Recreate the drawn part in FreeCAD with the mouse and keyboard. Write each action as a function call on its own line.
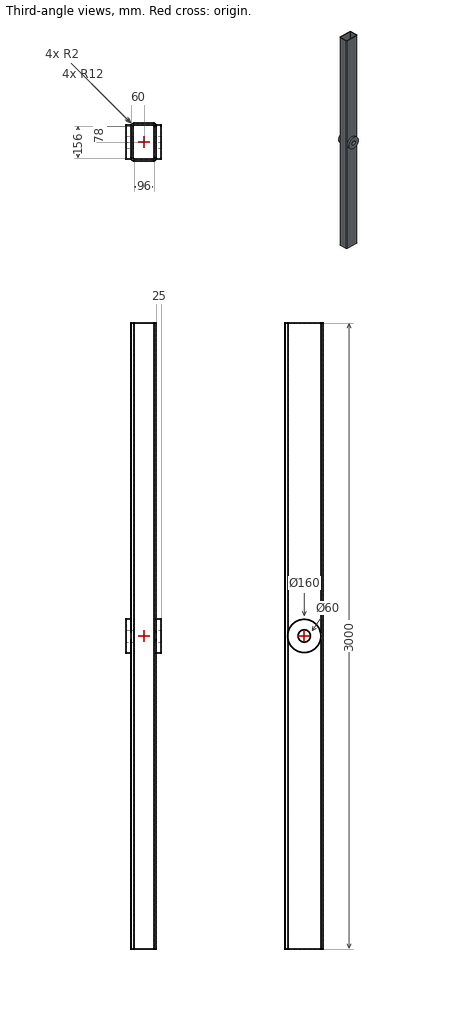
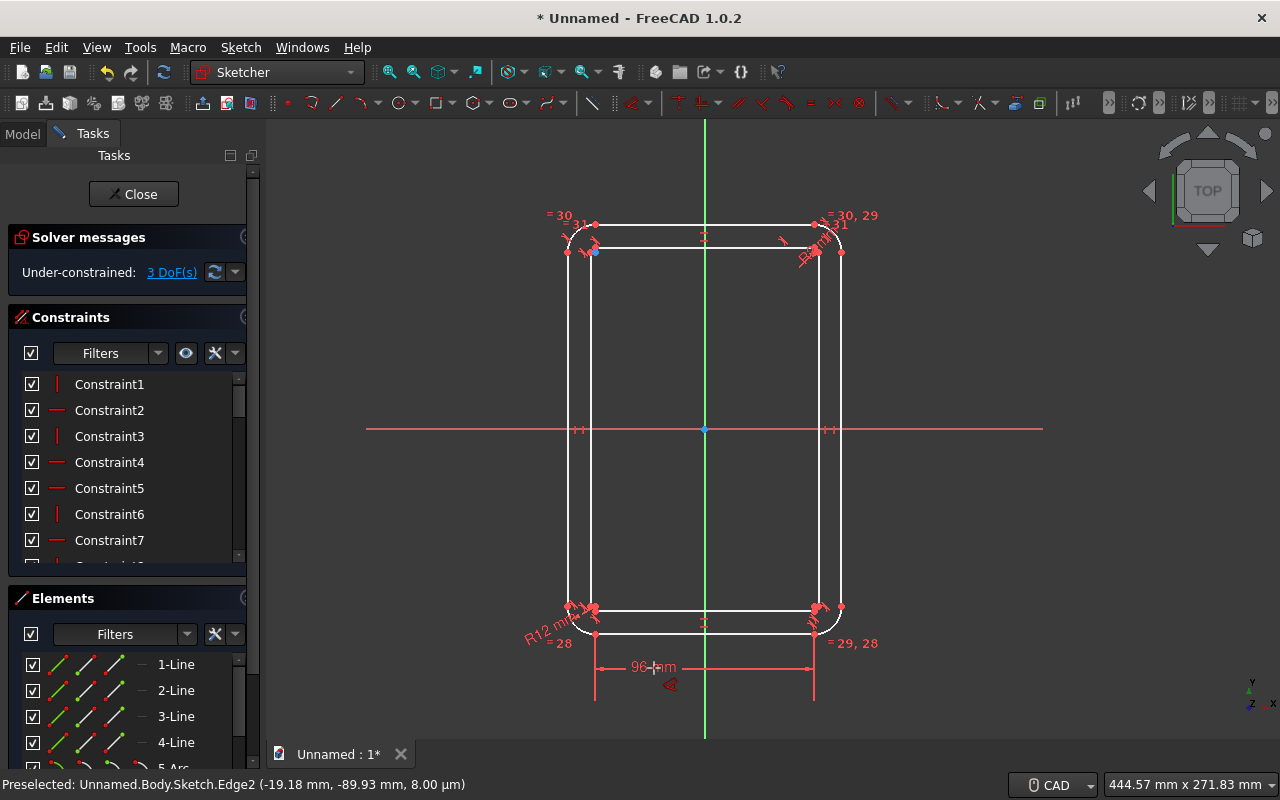
click(568, 359)
click(534, 348)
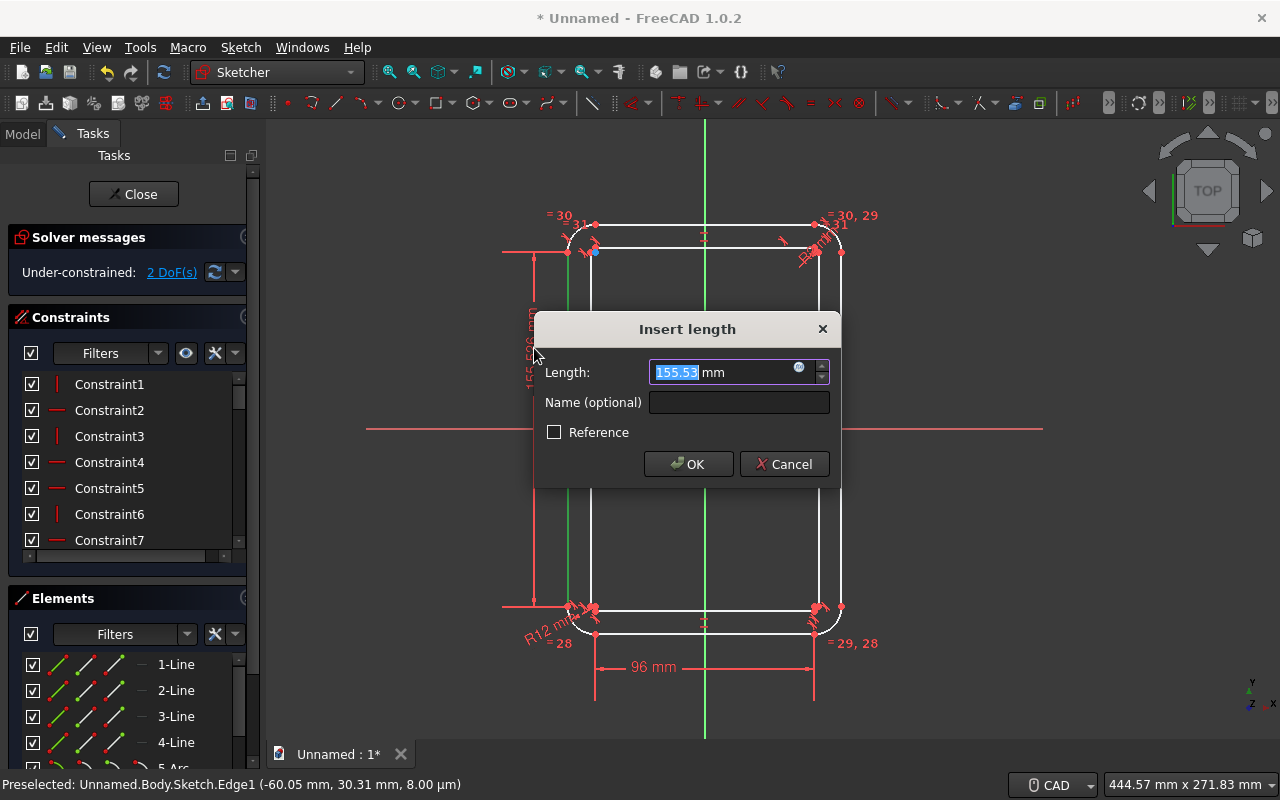
text(156)
key(Return)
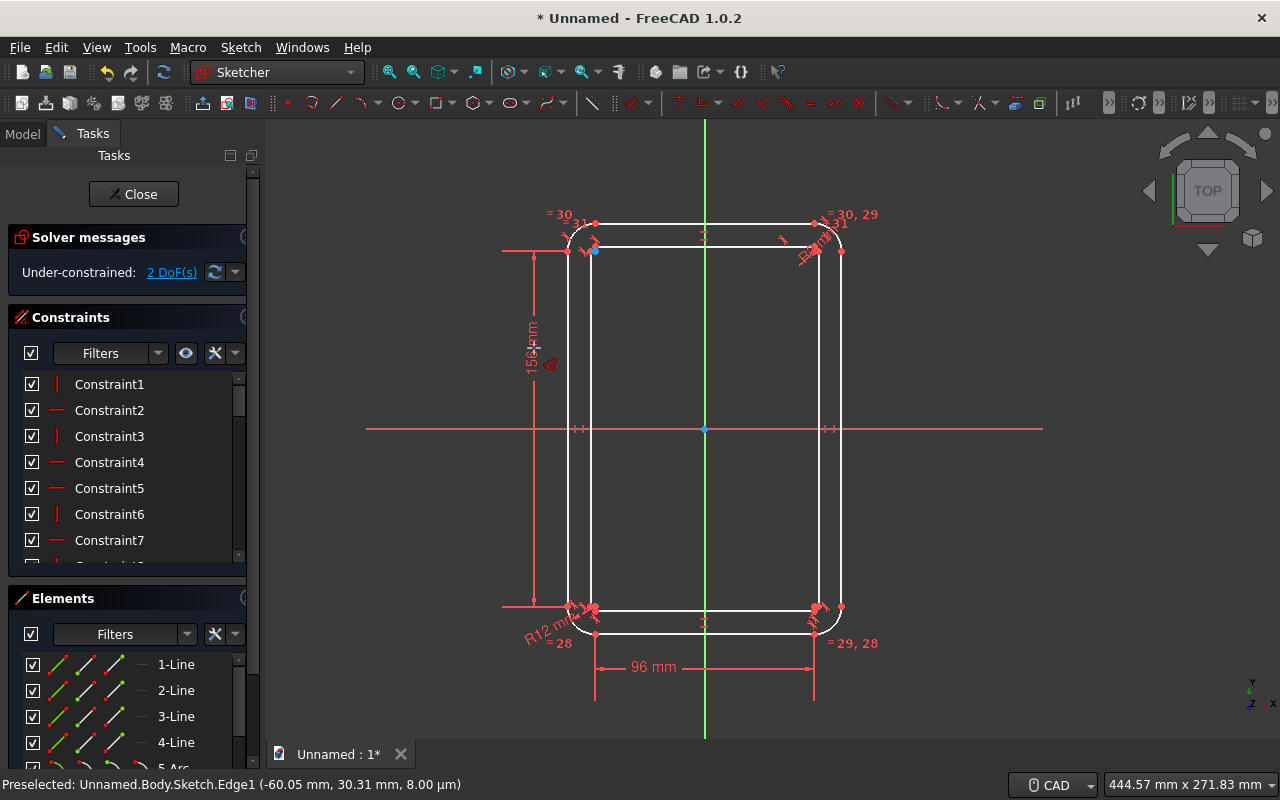
click(568, 251)
click(636, 463)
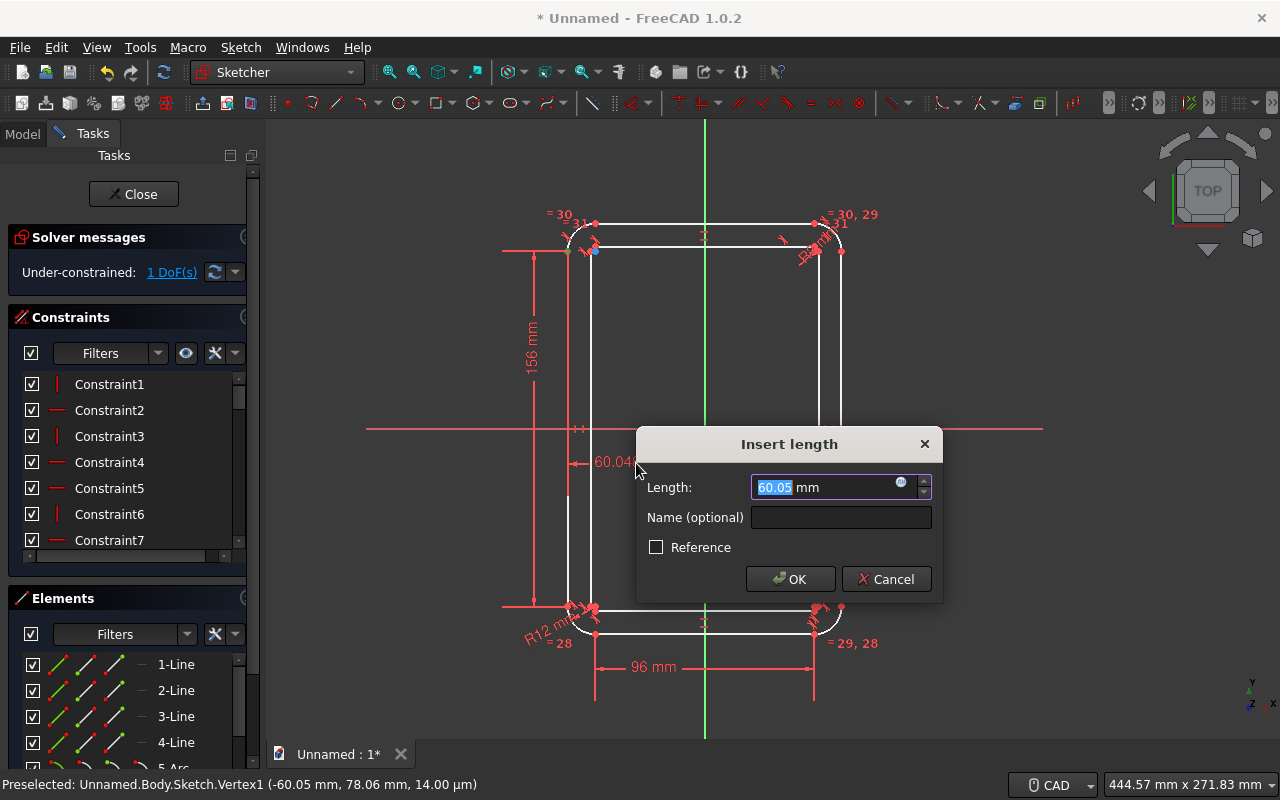
text(60)
key(Return)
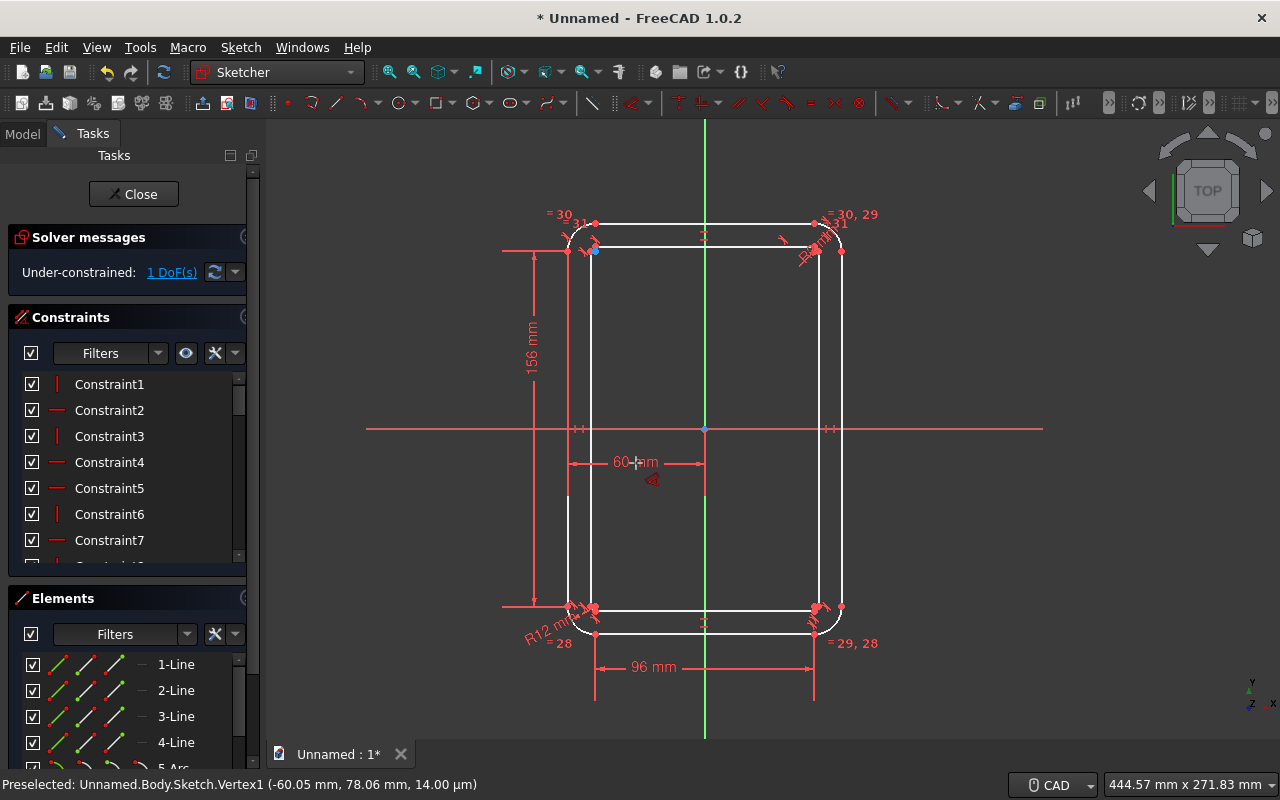
click(568, 251)
click(534, 299)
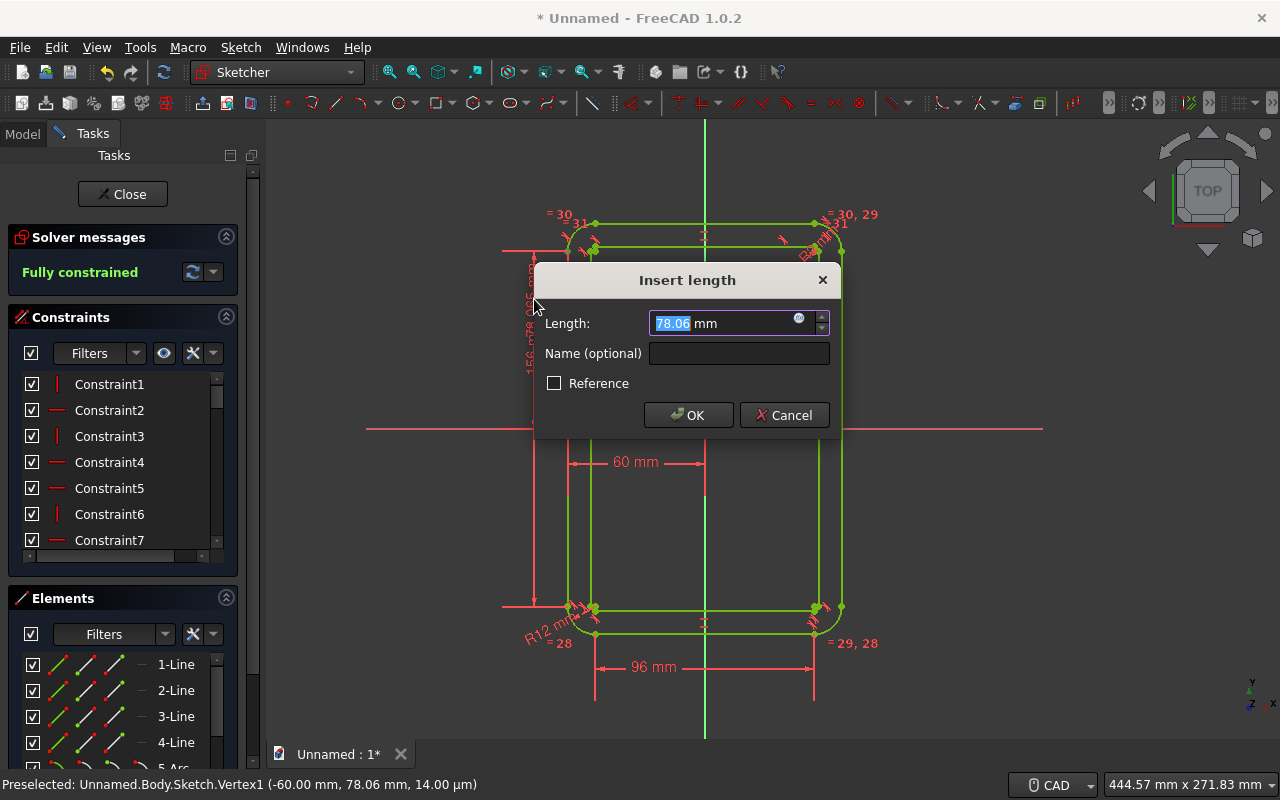
text(78)
key(Return)
key(Escape)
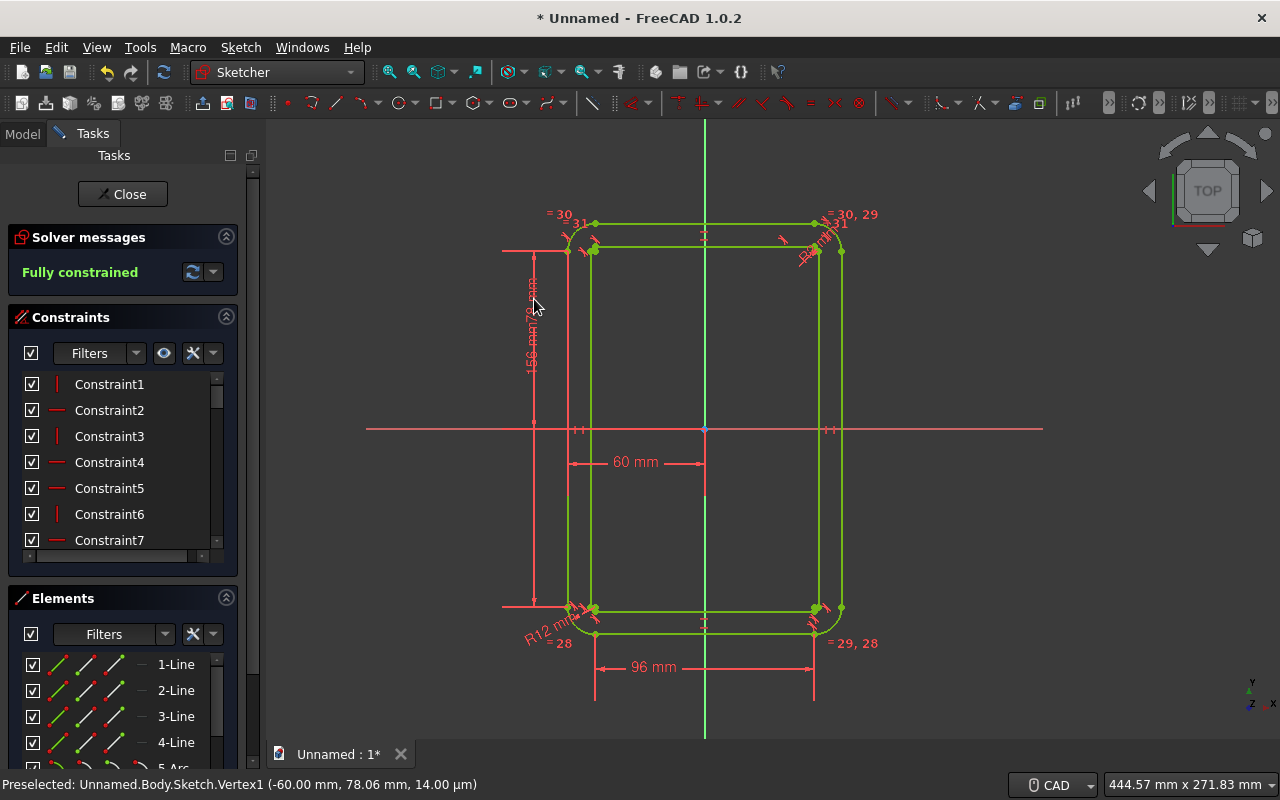
click(123, 194)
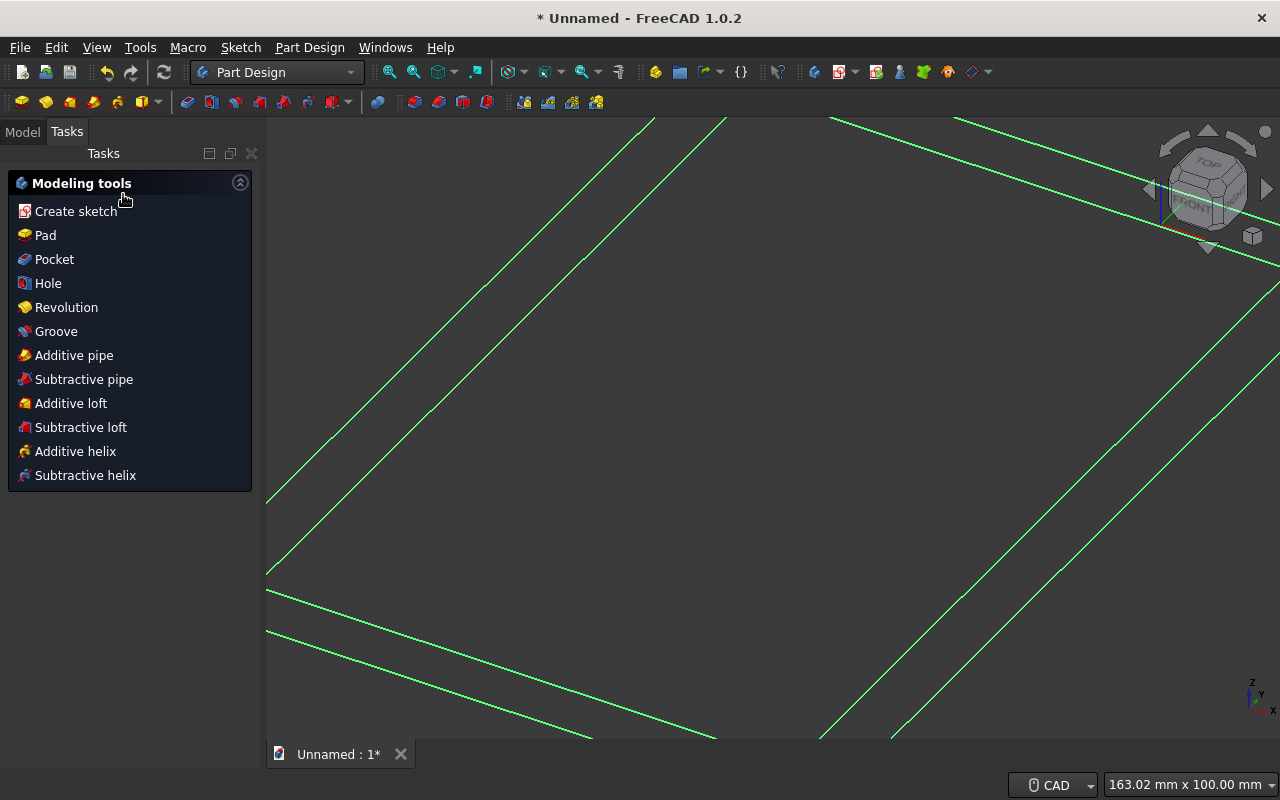
click(22, 102)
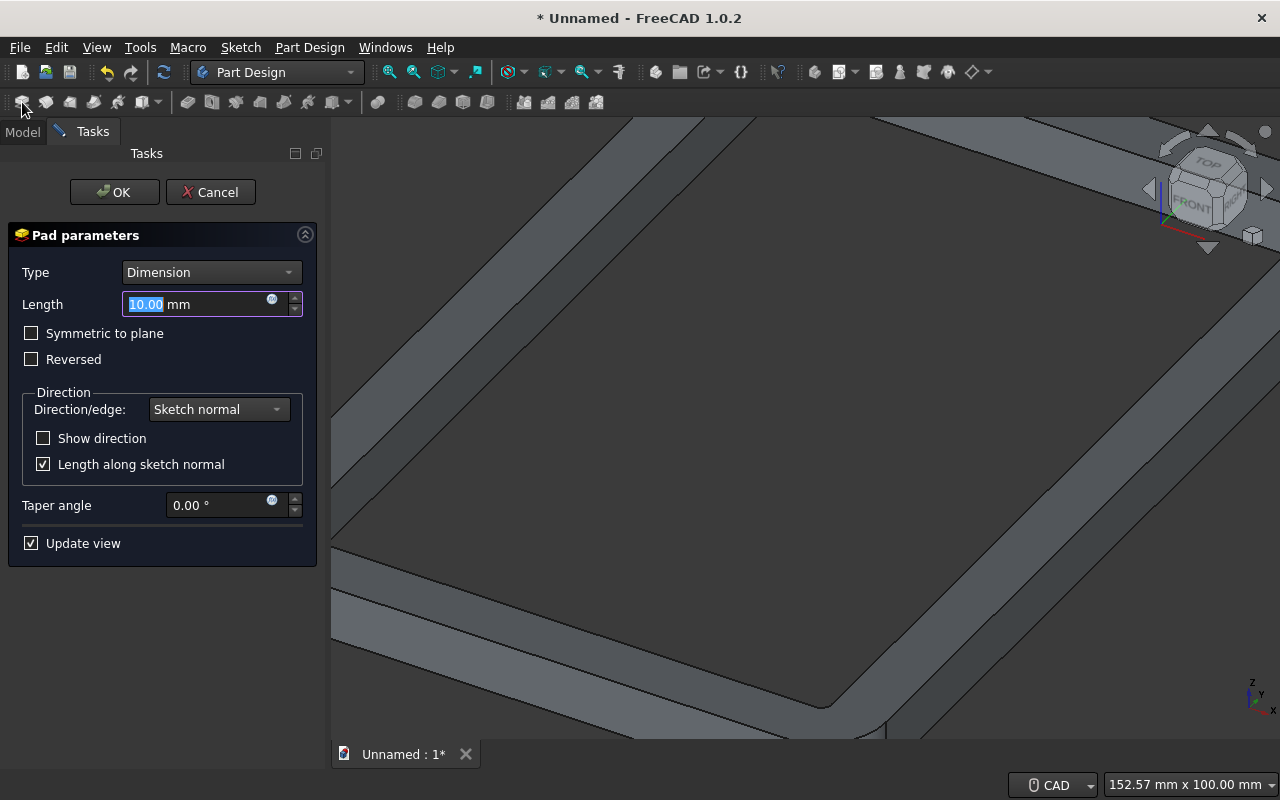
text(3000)
key(Tab)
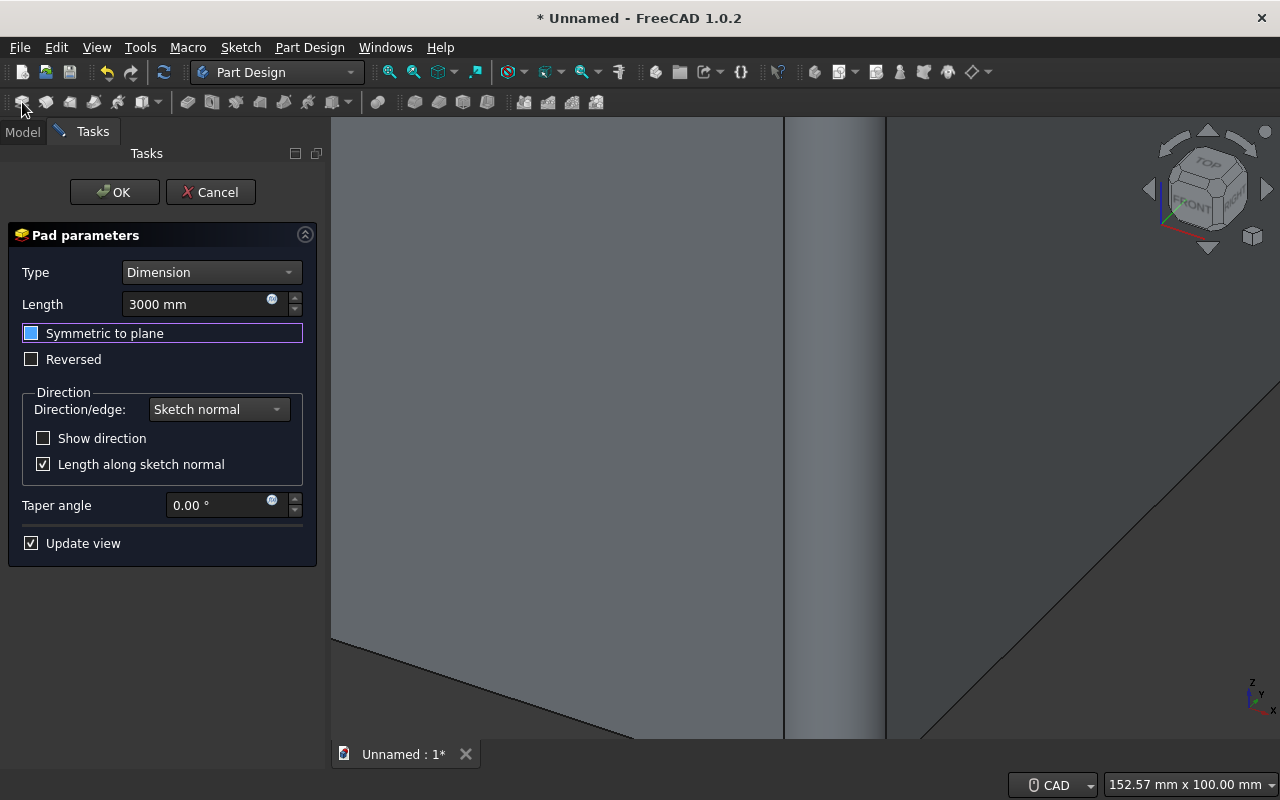
click(30, 333)